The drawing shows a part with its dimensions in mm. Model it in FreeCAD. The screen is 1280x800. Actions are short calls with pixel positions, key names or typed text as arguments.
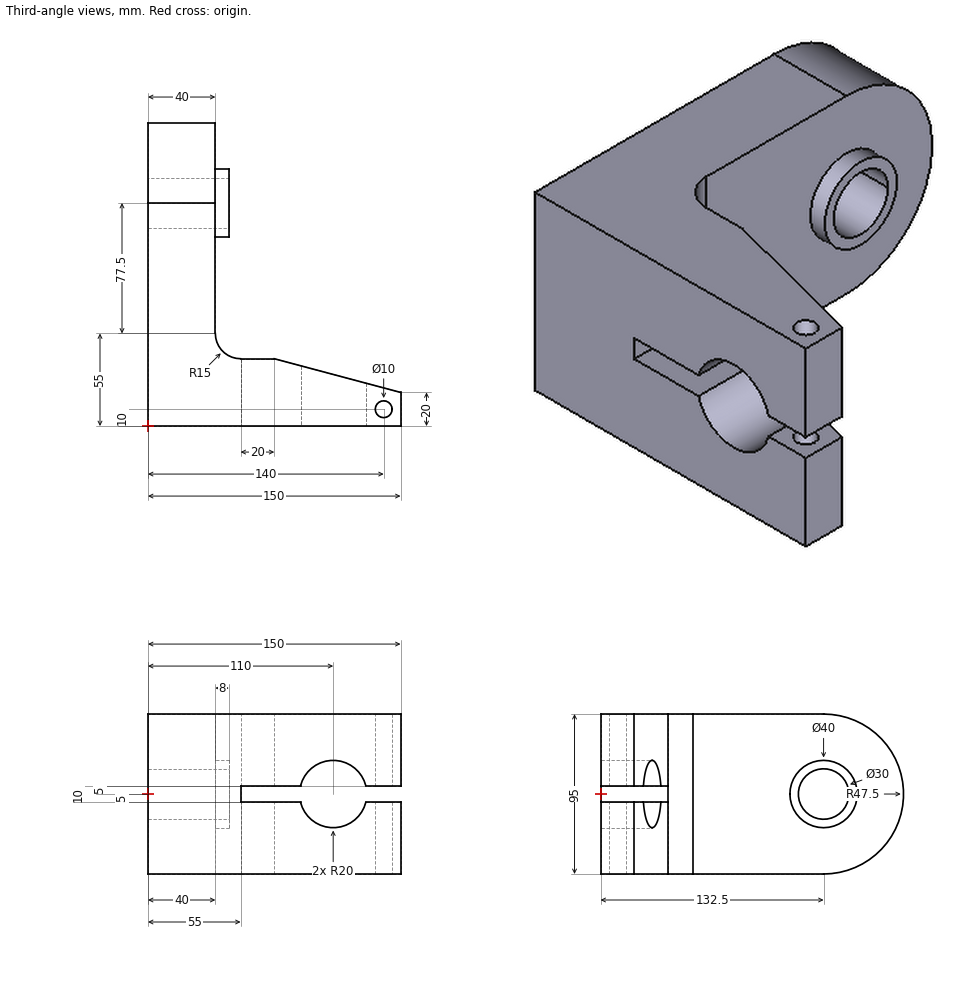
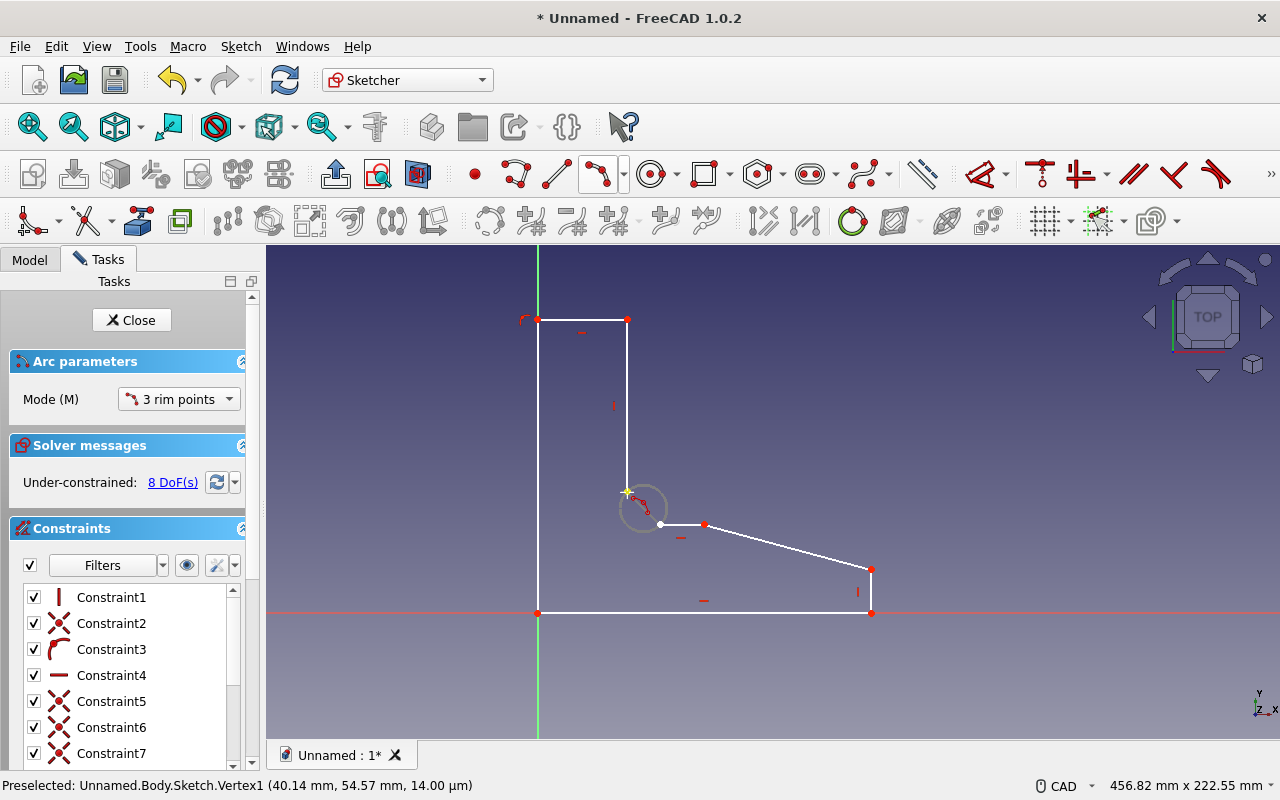
scroll(636, 515, up, 3)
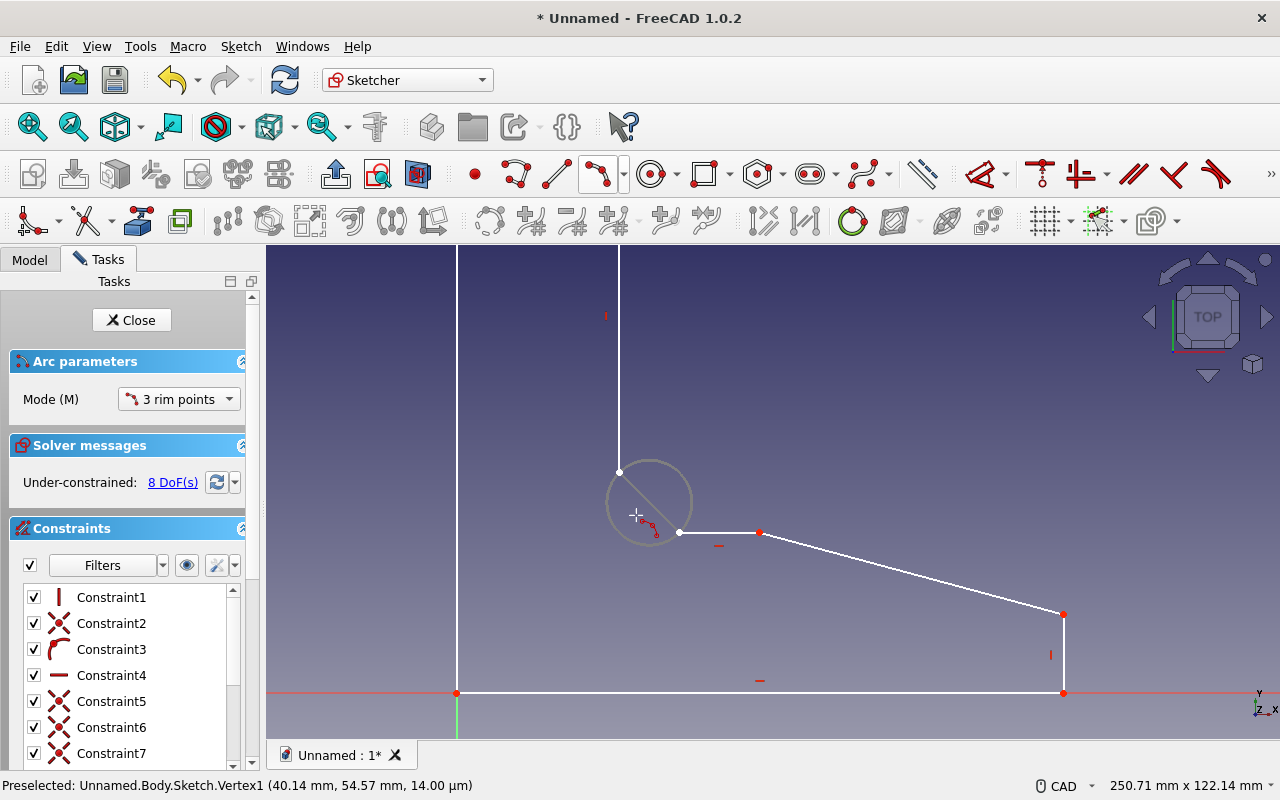
click(637, 514)
key(Escape)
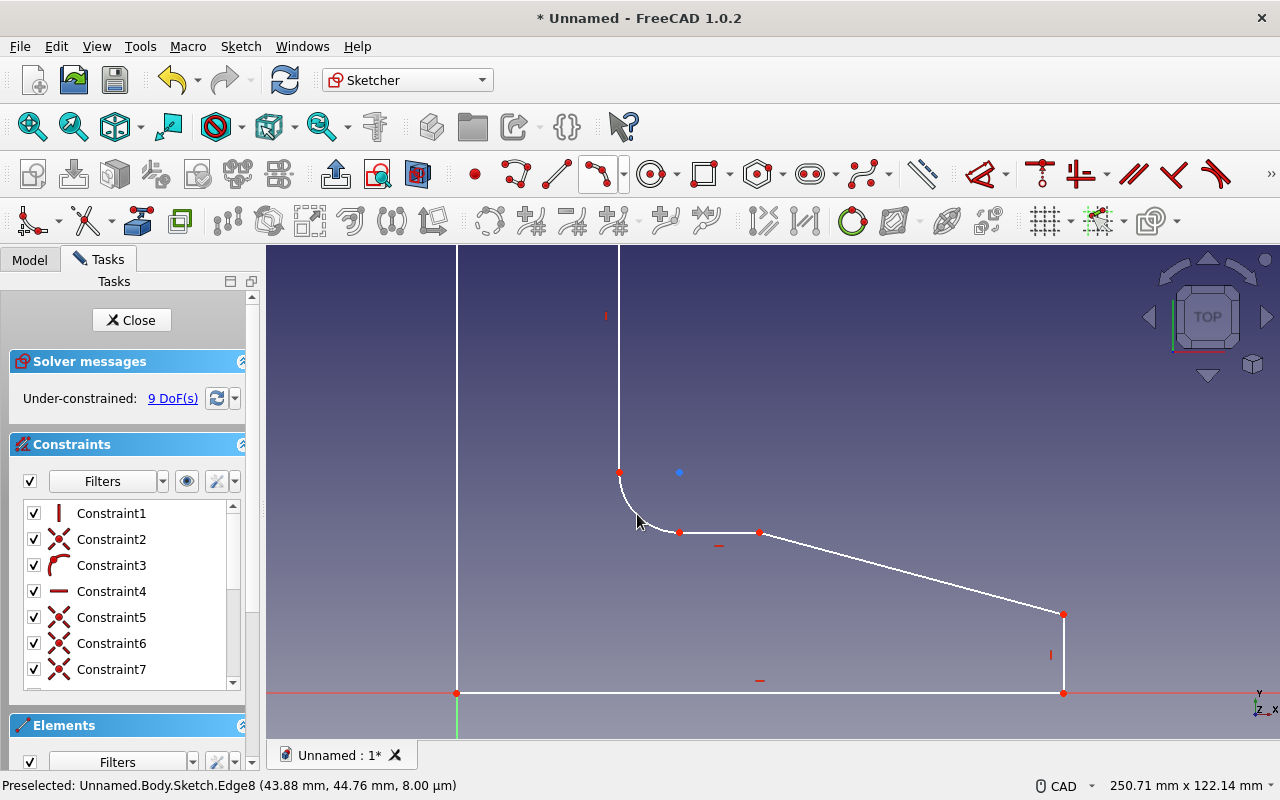
click(619, 379)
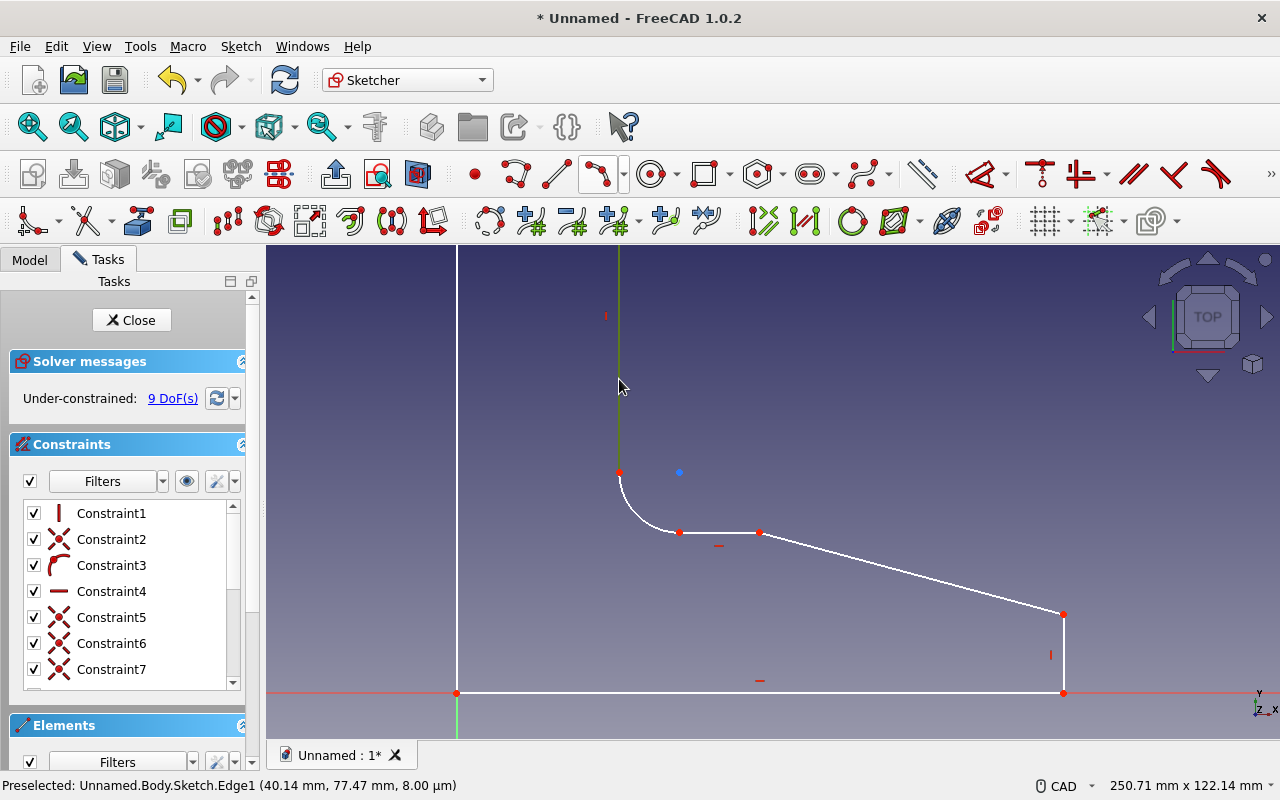
click(626, 500)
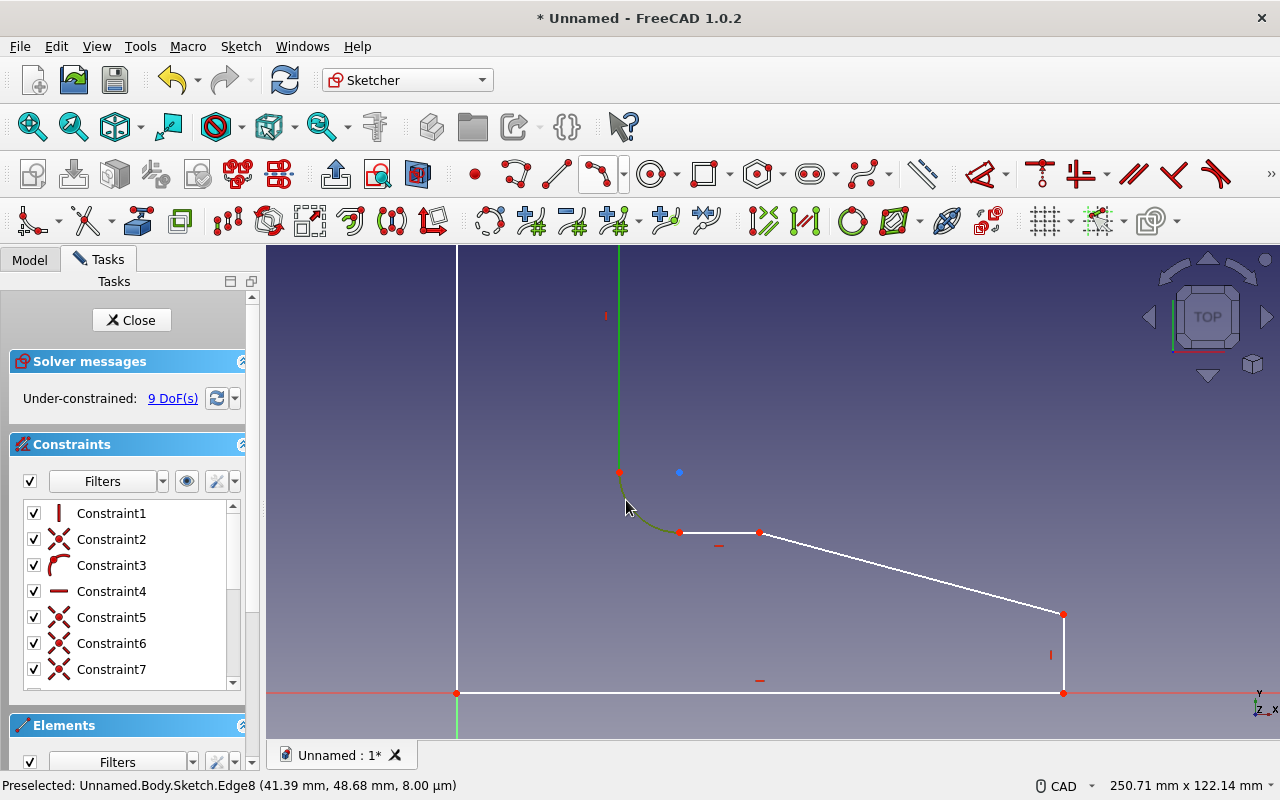
click(1216, 174)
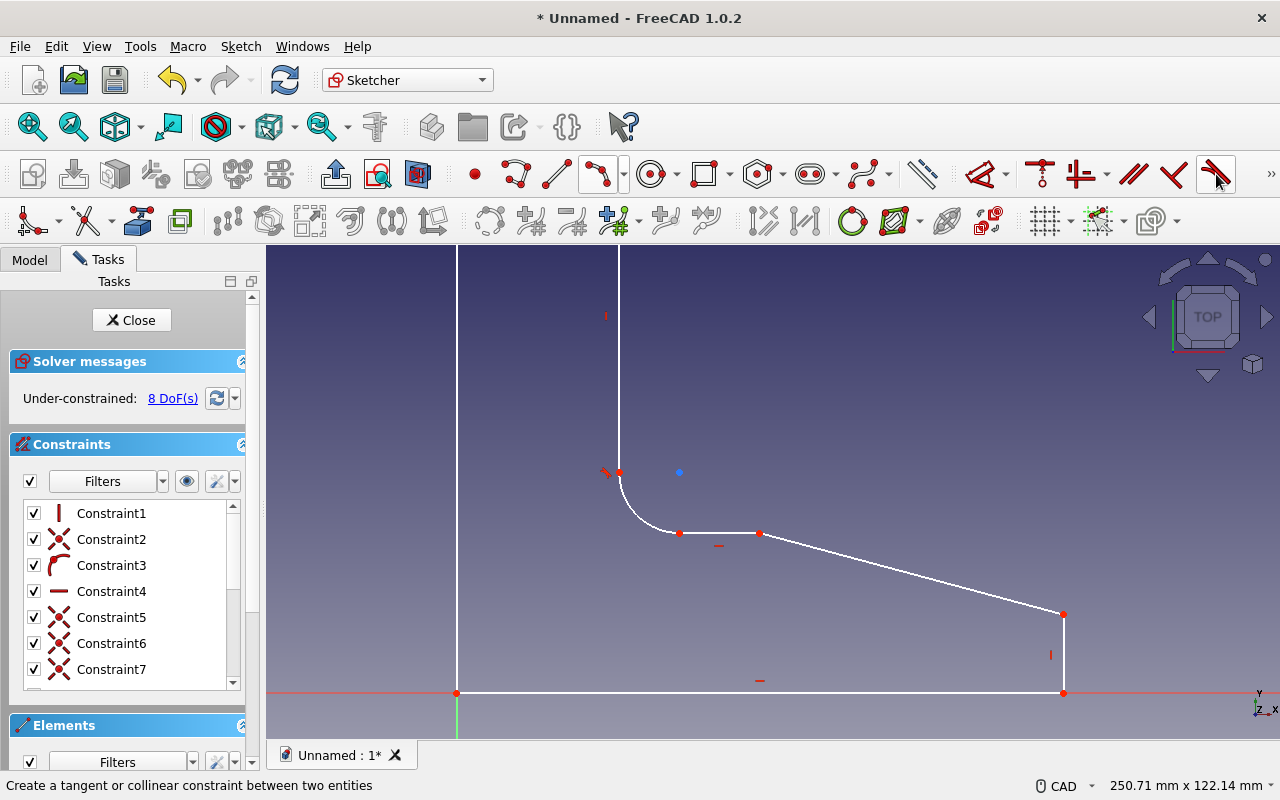
click(736, 533)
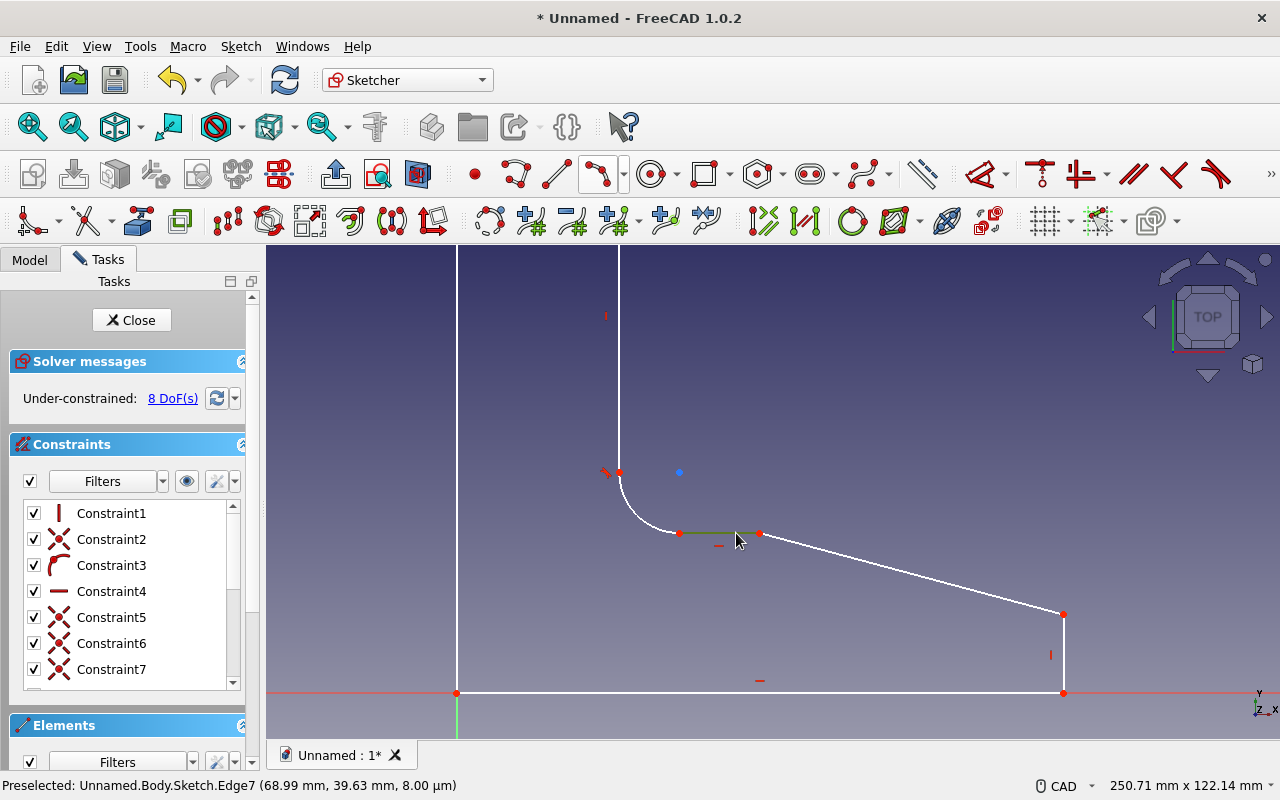
click(626, 500)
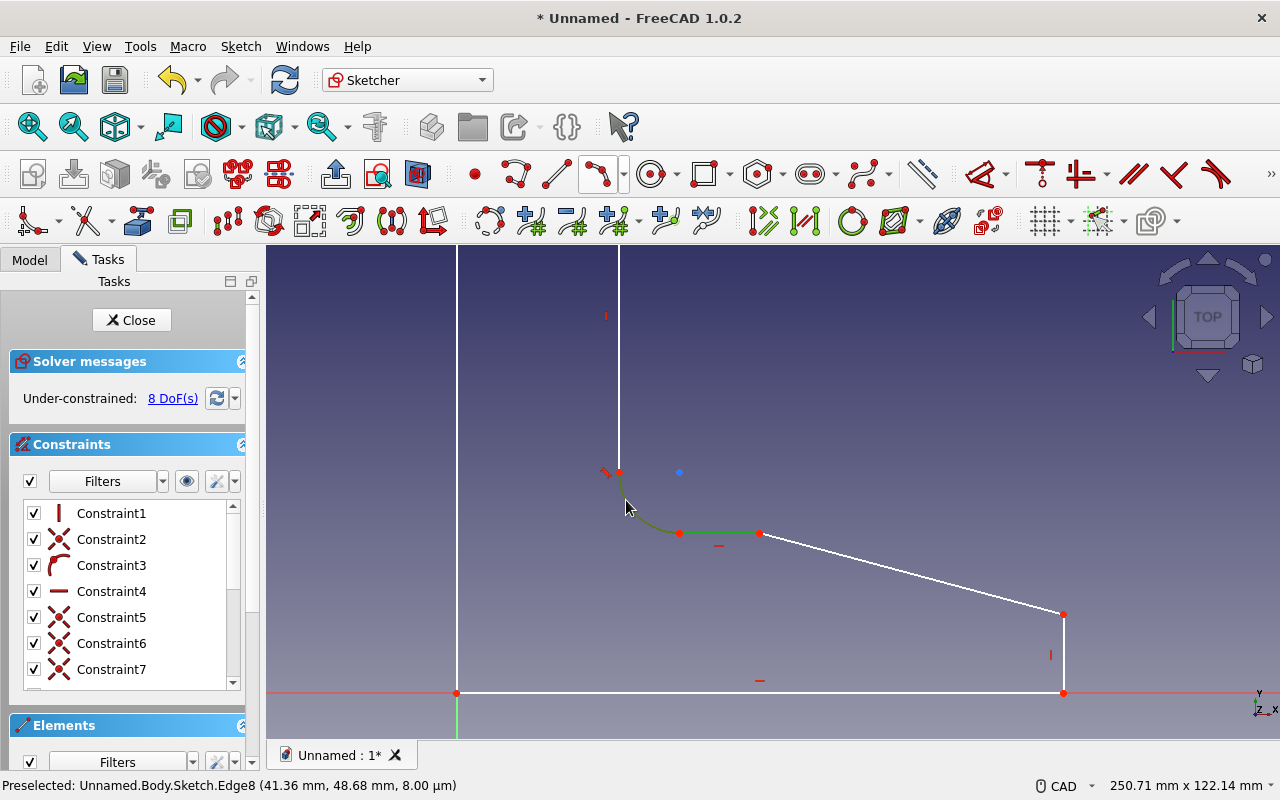
click(1216, 174)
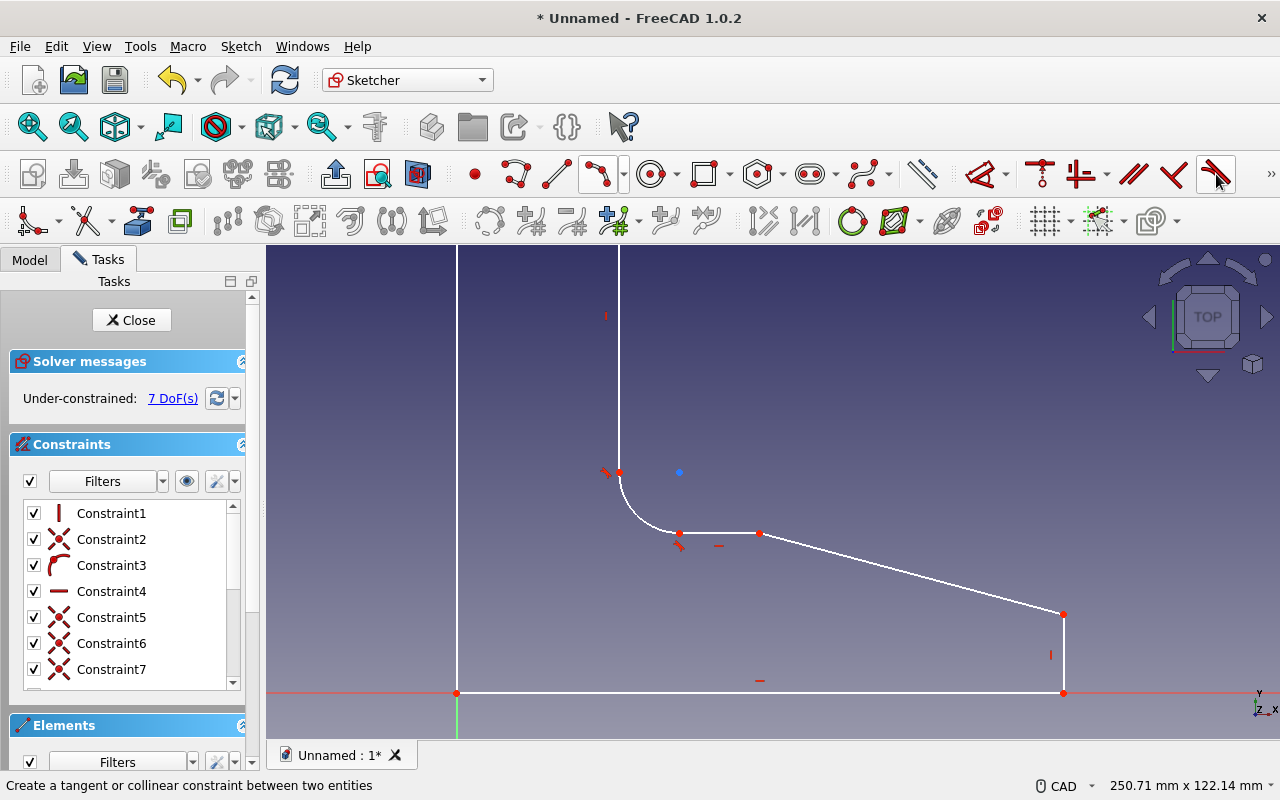
click(980, 174)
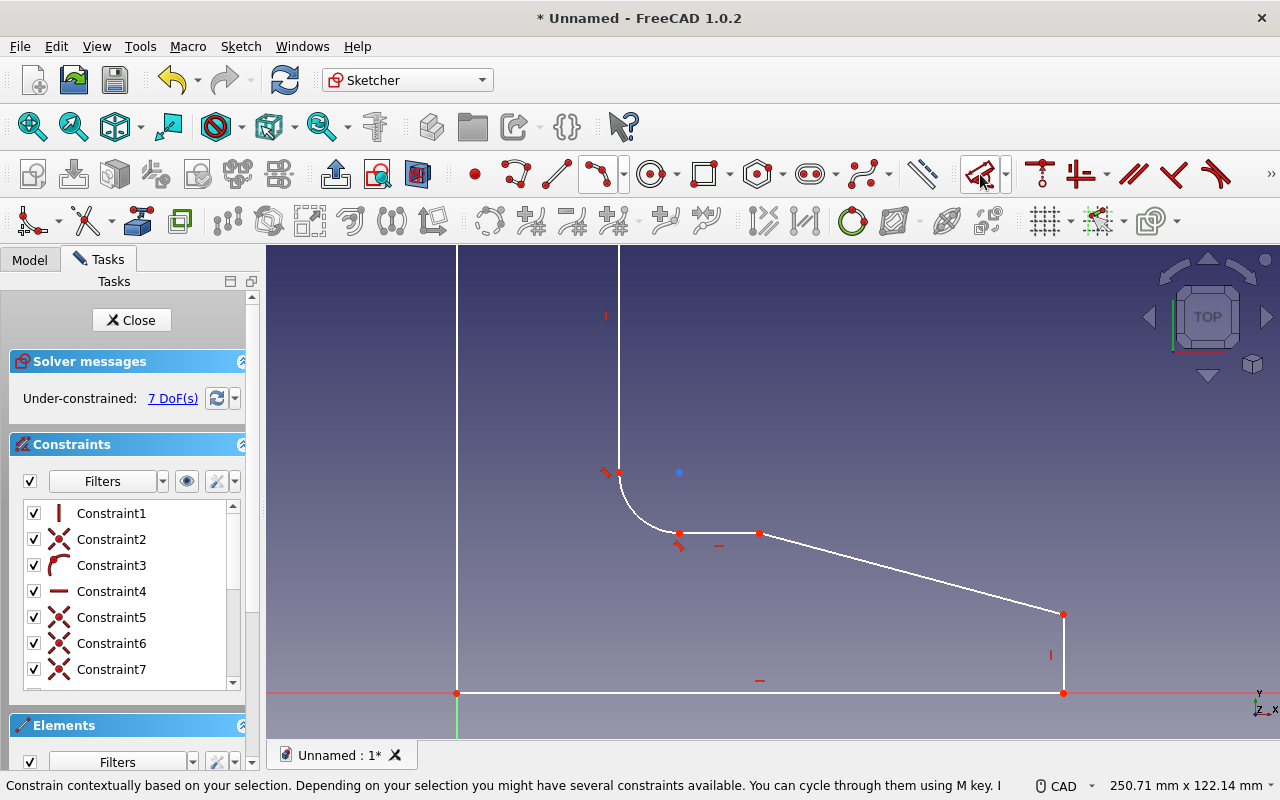
click(626, 500)
click(597, 515)